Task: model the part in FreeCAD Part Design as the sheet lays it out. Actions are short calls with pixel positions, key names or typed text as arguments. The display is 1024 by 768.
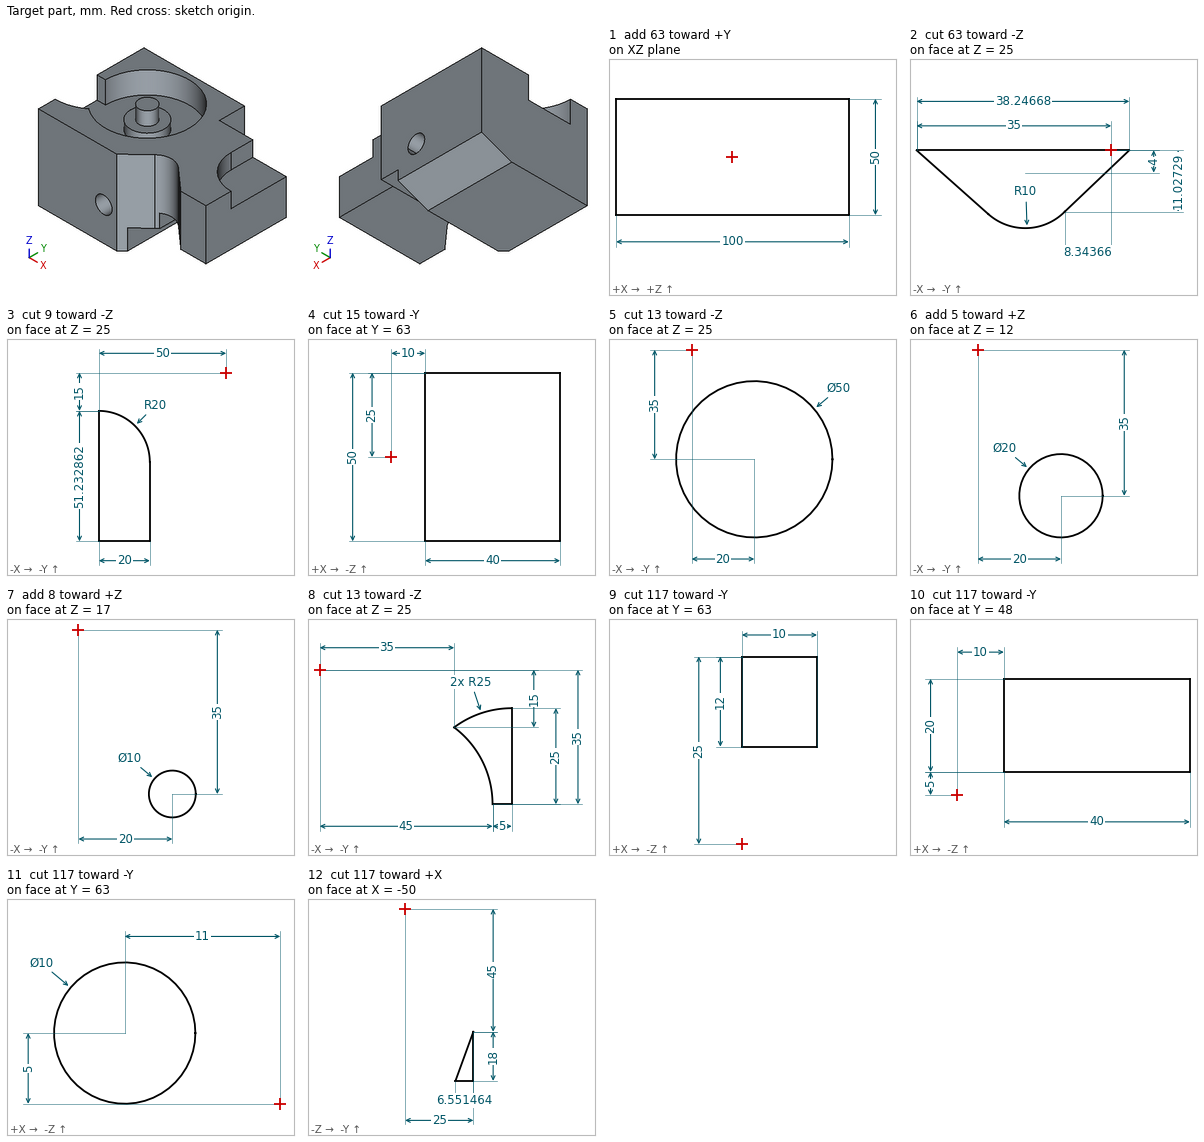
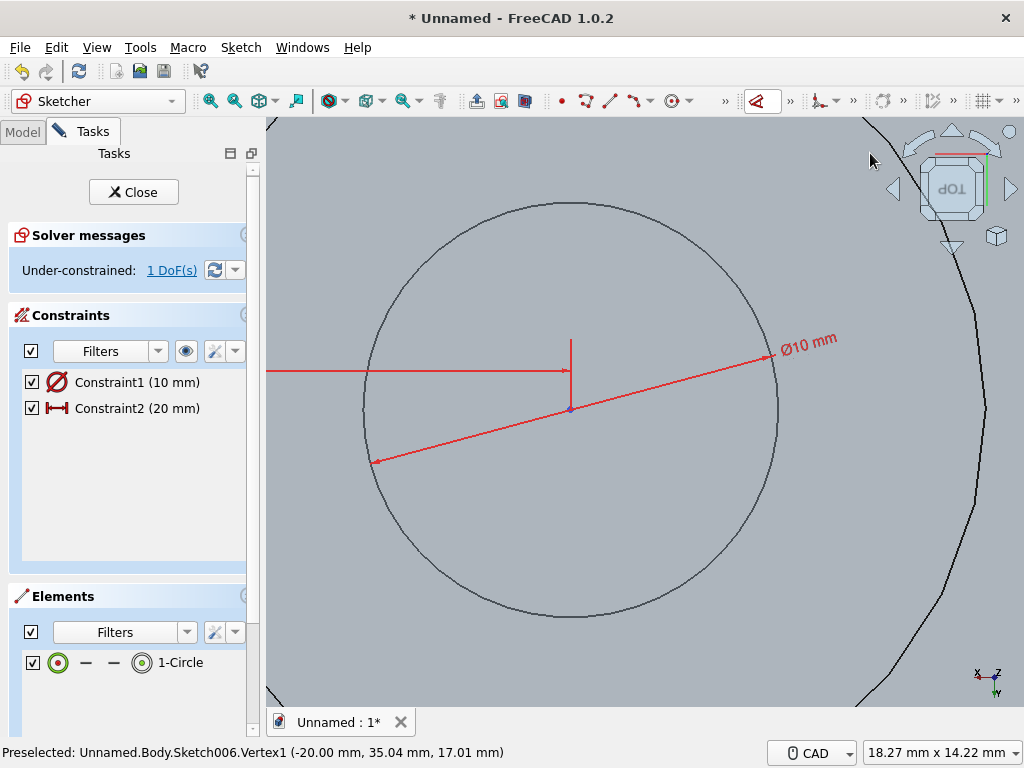
click(571, 410)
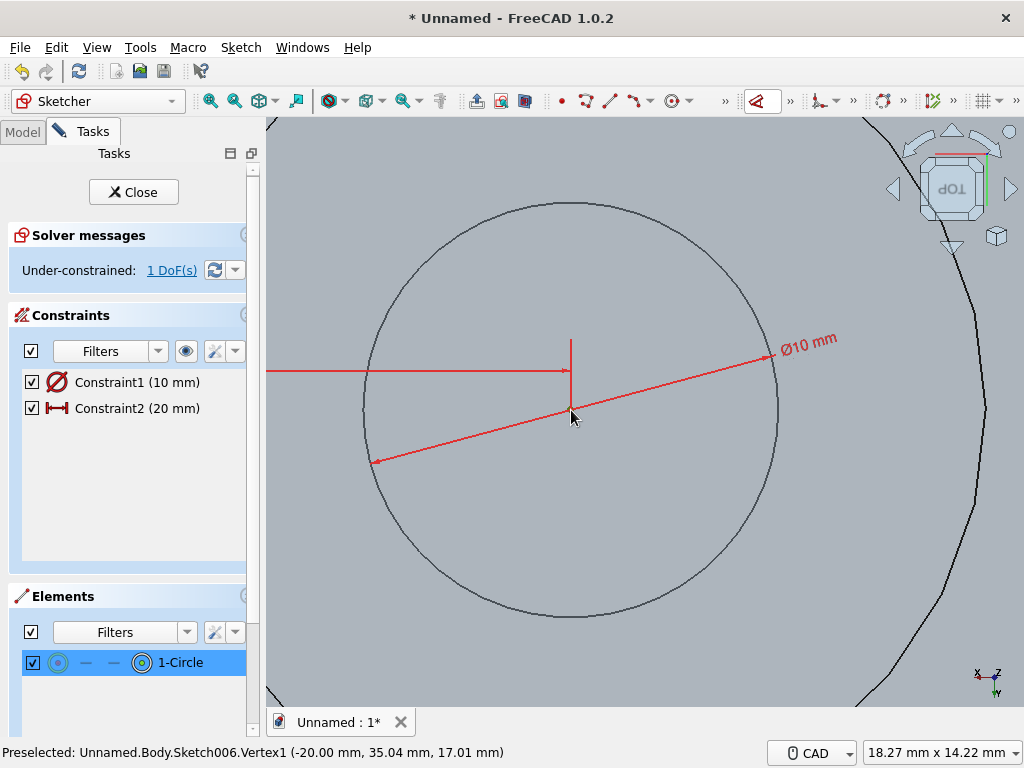
click(776, 102)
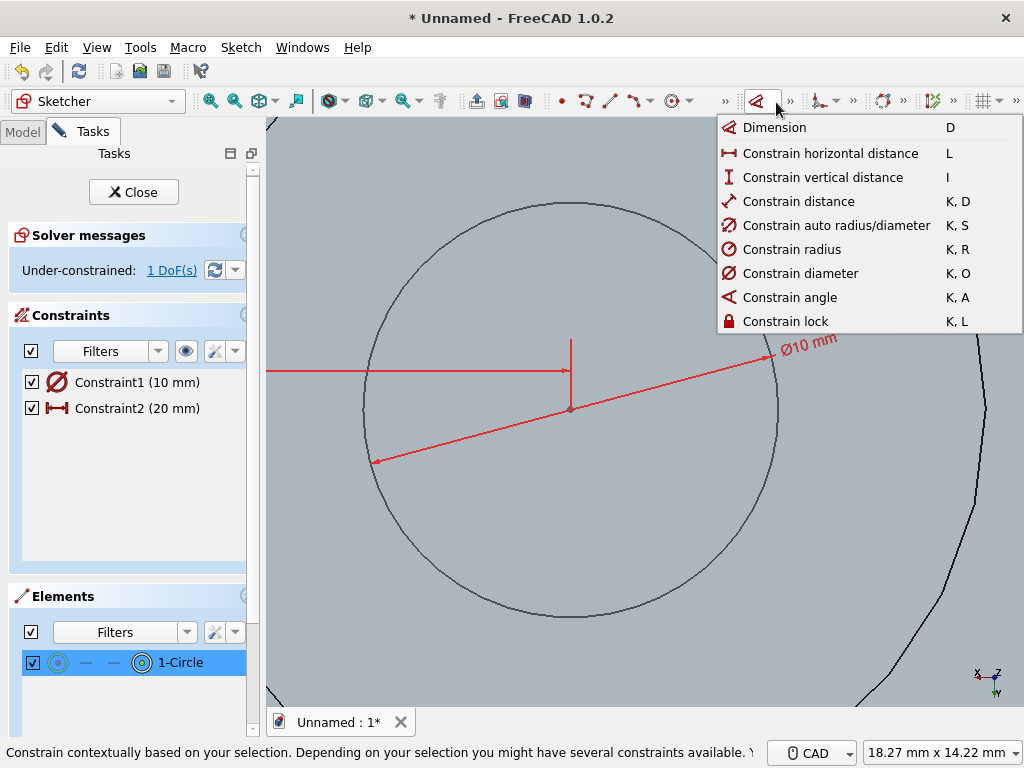
click(870, 177)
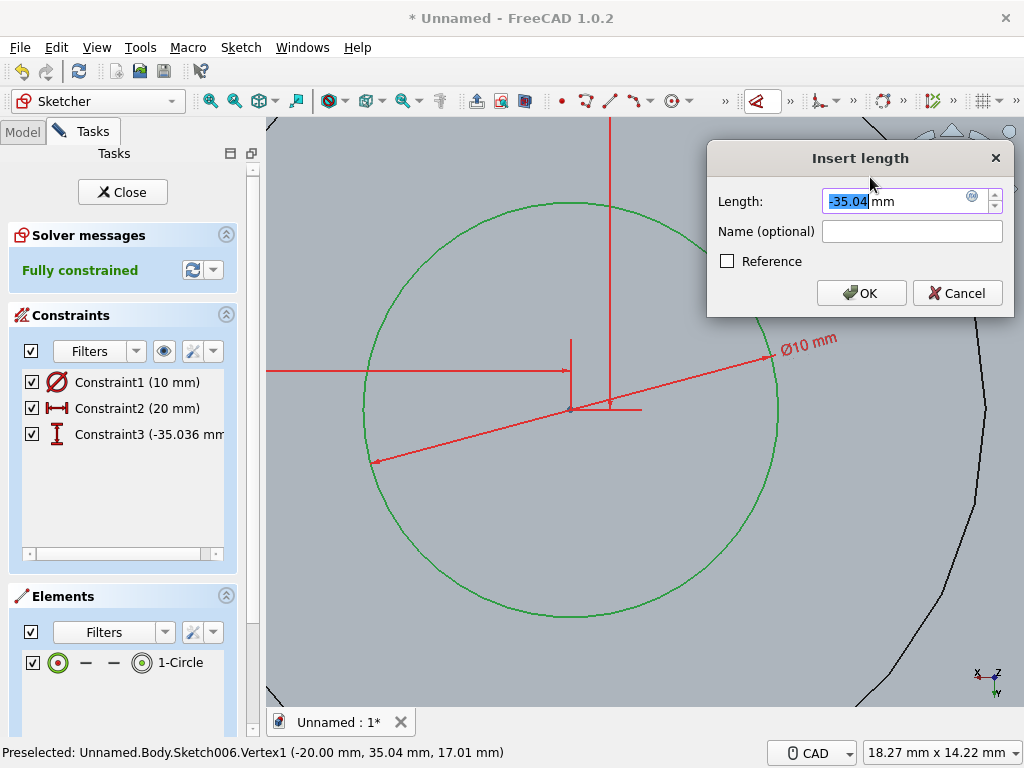
text(-35)
key(Return)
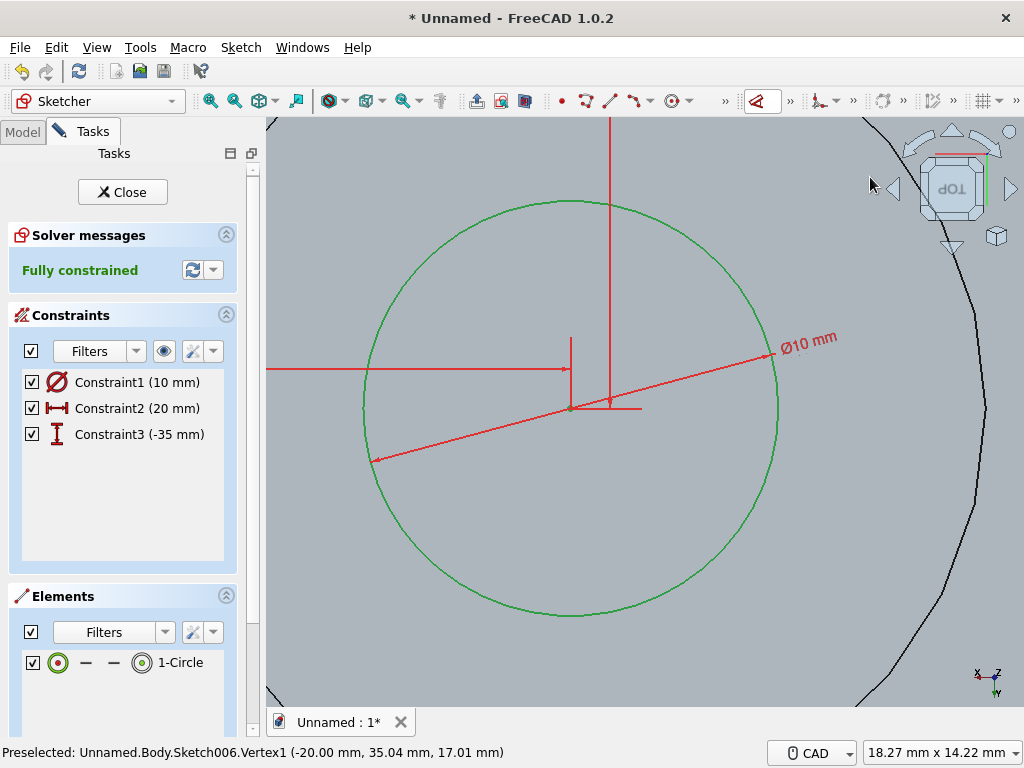
click(123, 192)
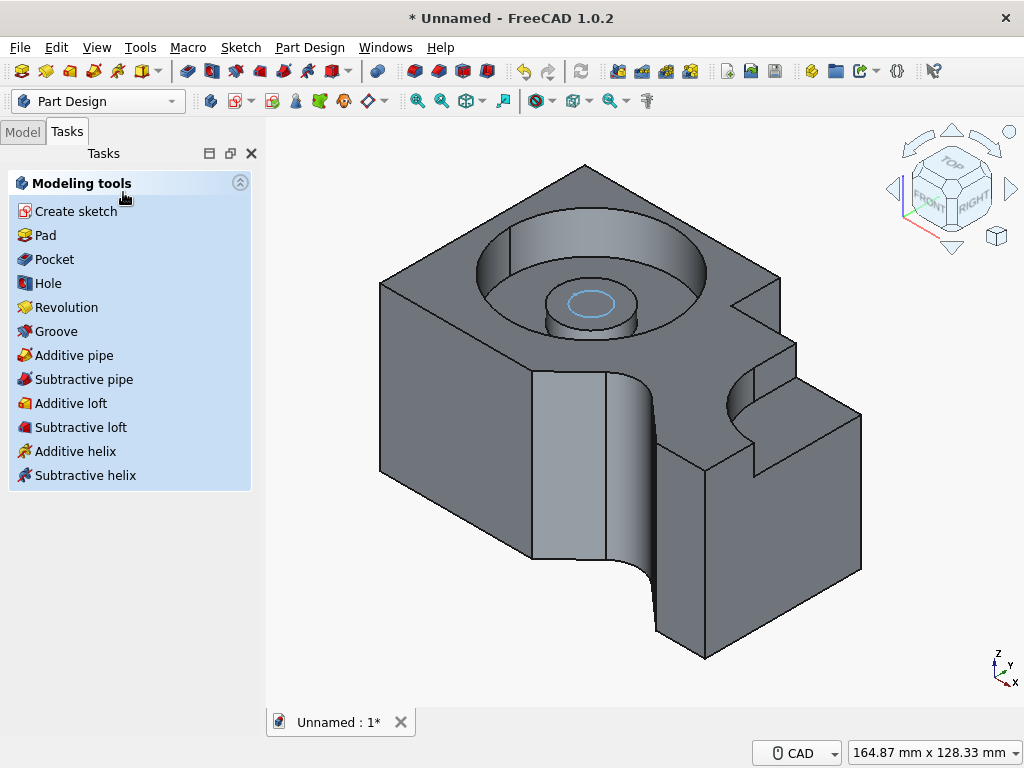
click(22, 72)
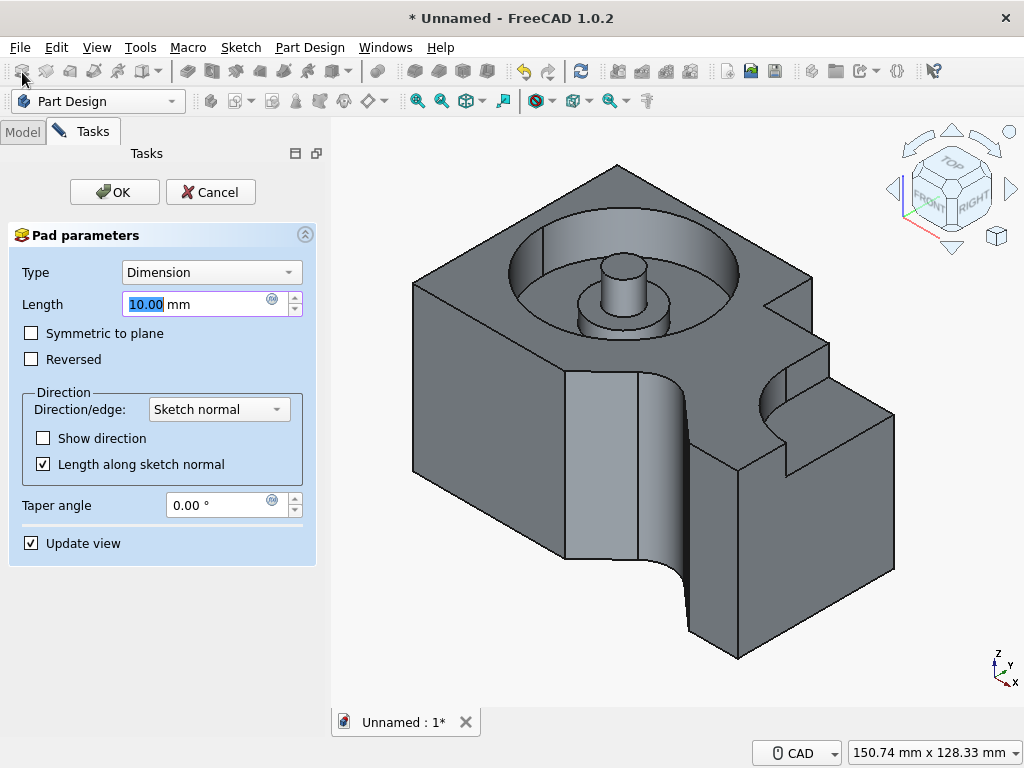
text(8)
key(Tab)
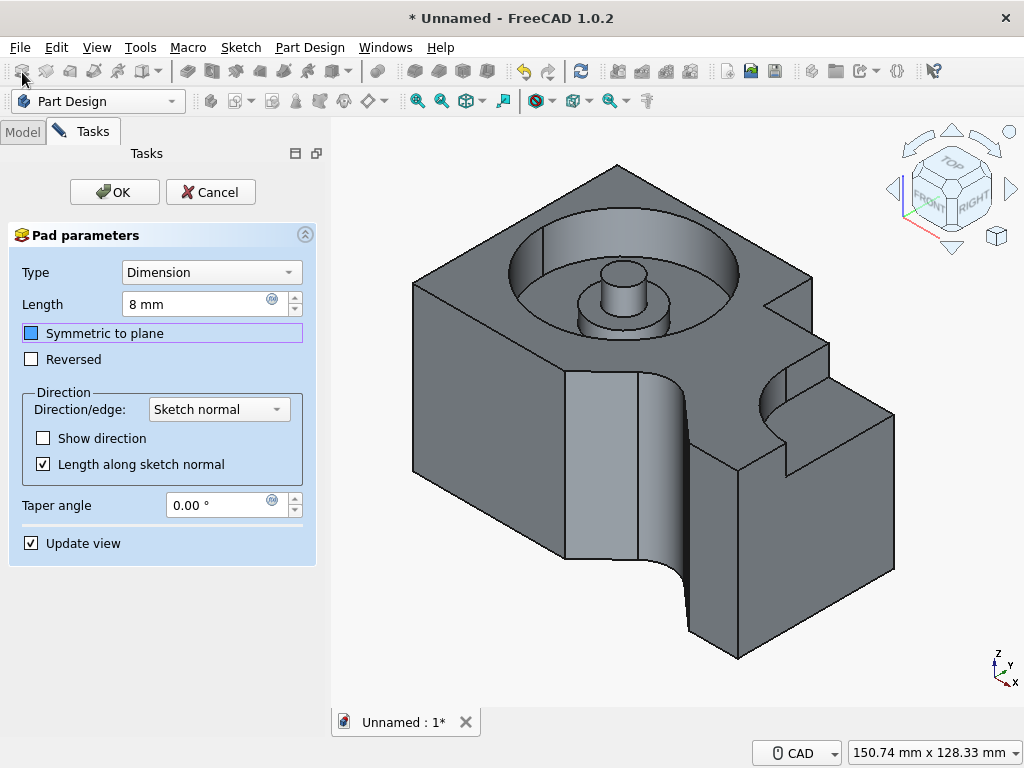
click(115, 192)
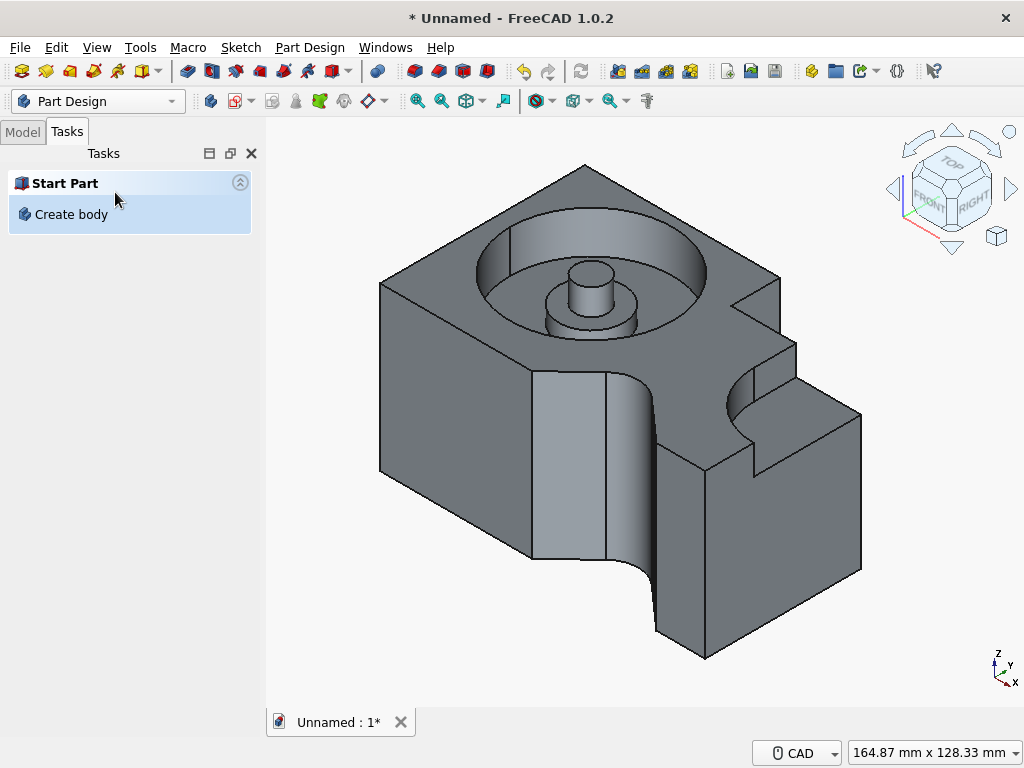
click(691, 344)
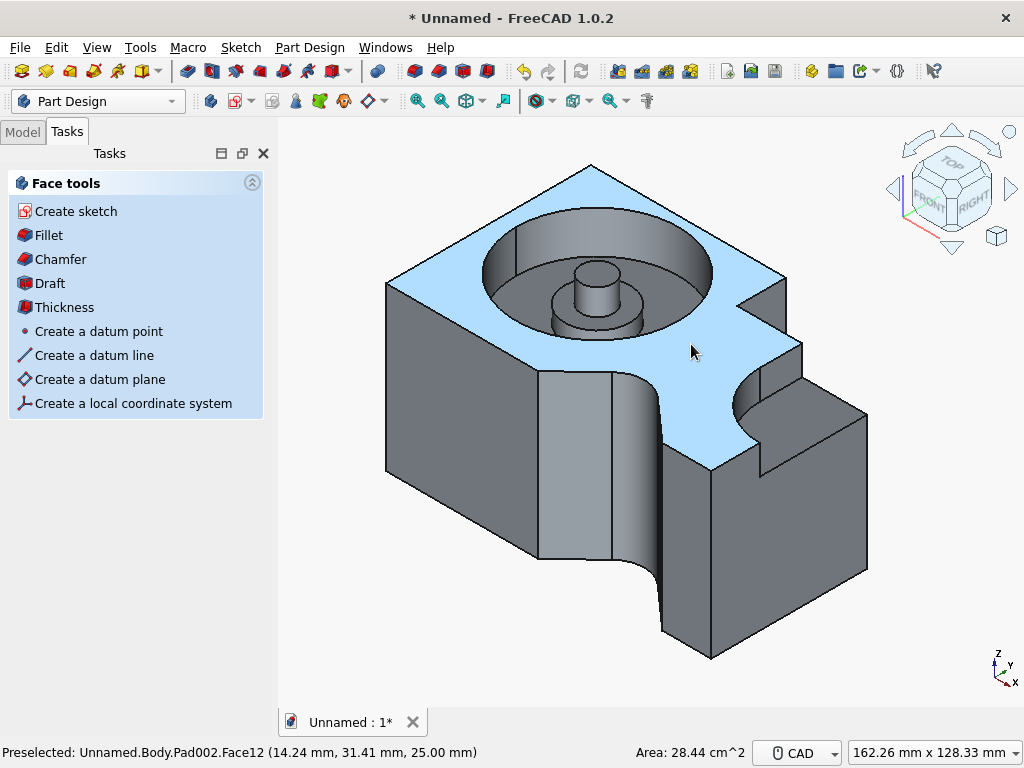
click(236, 102)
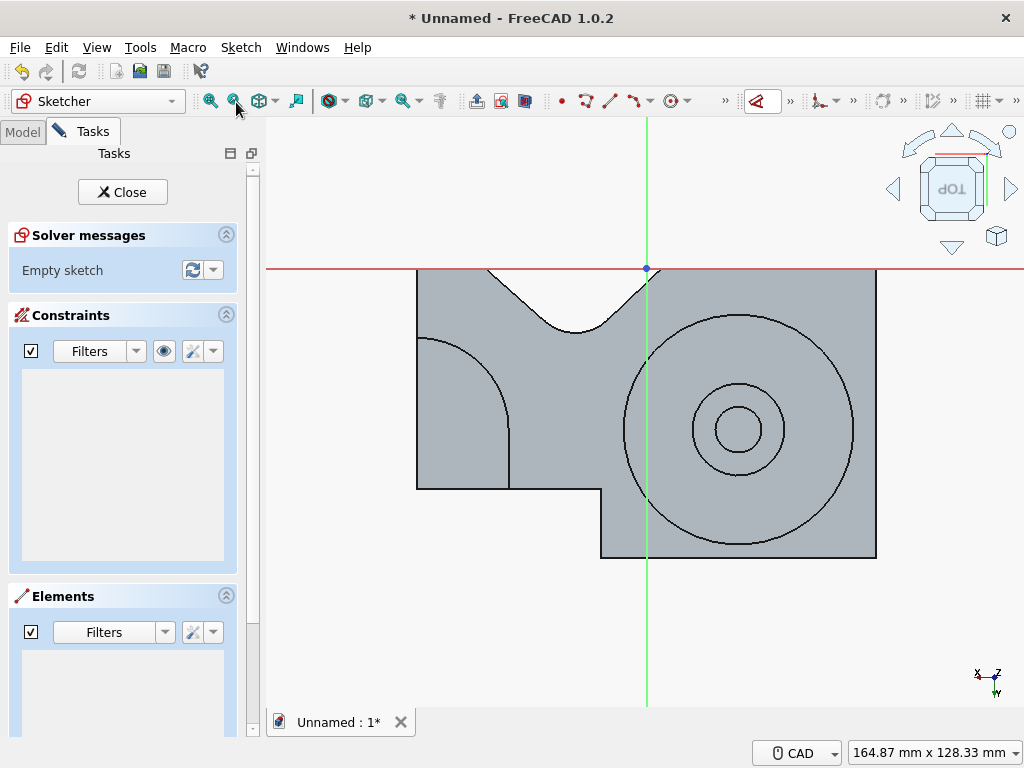
scroll(576, 412, down, 5)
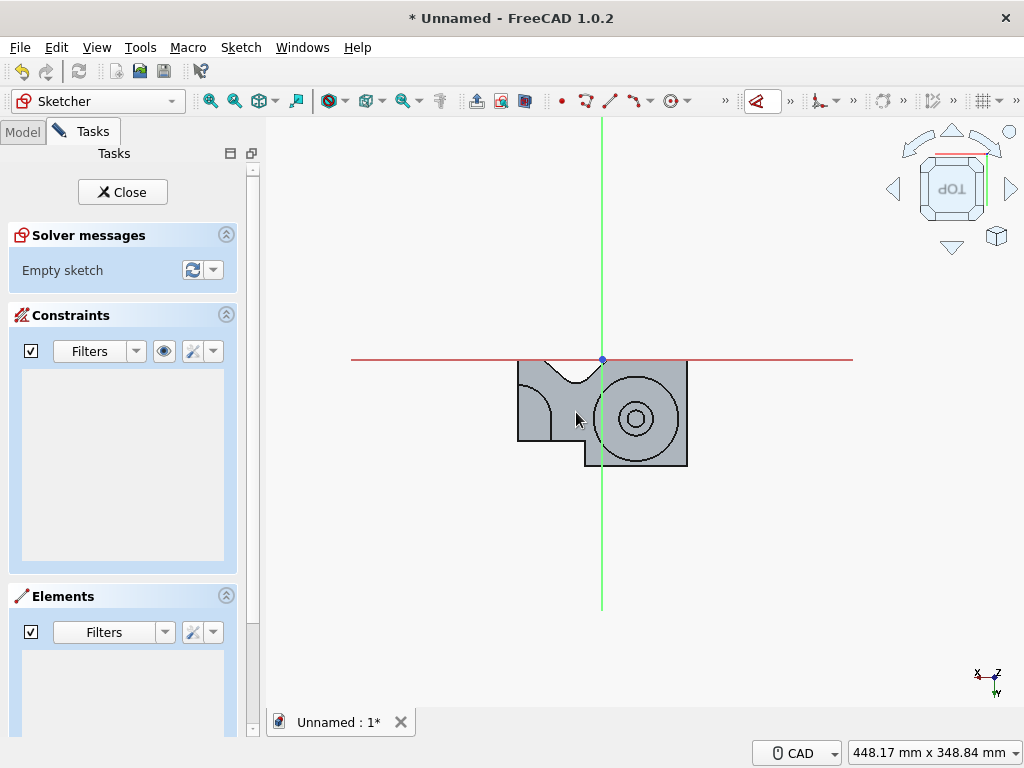
scroll(662, 383, up, 8)